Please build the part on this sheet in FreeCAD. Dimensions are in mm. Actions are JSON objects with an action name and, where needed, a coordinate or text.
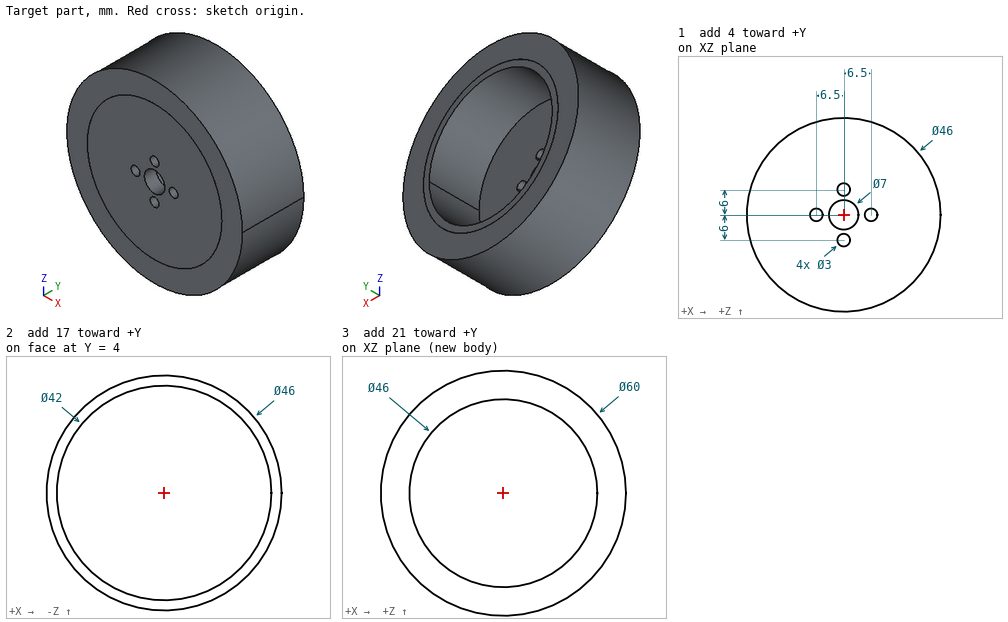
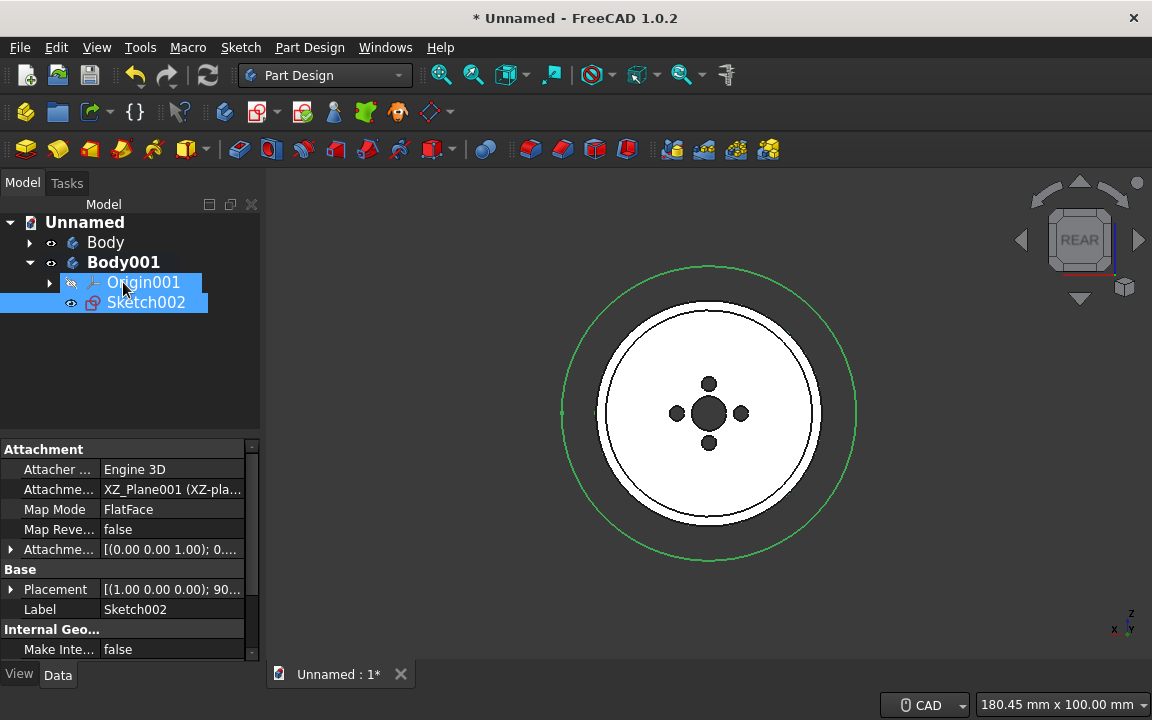
{"action": "left_click", "coordinate": [26, 150]}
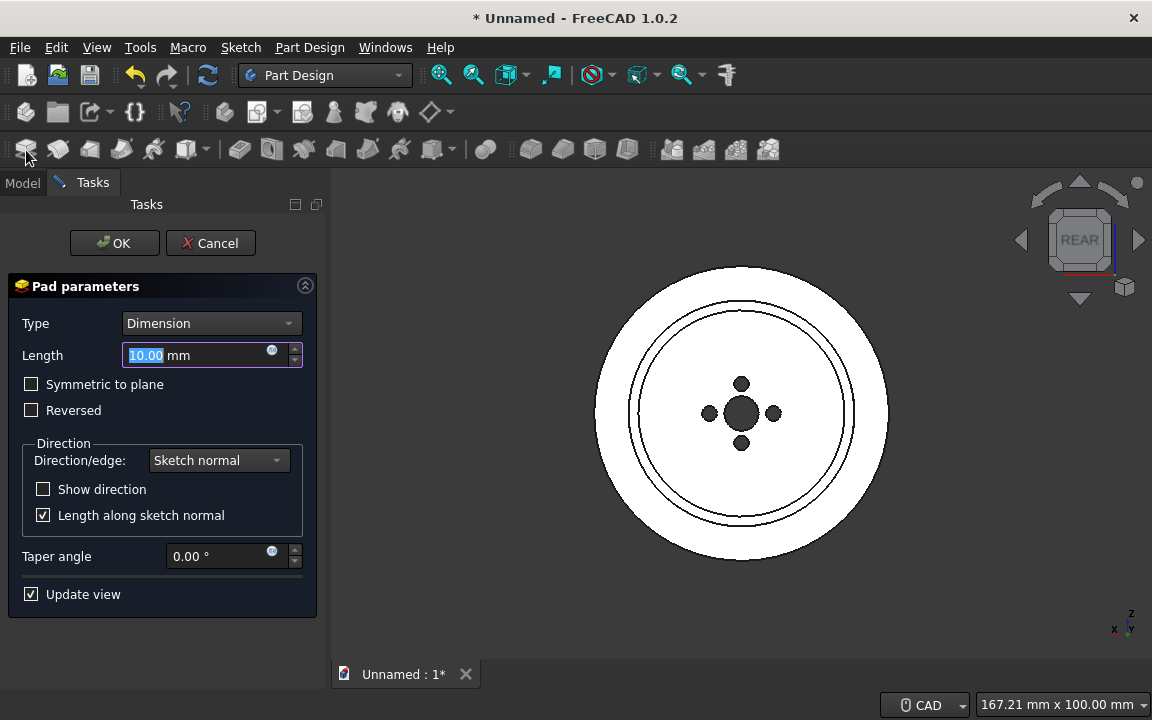
{"action": "type", "text": "21"}
{"action": "key", "text": "Tab"}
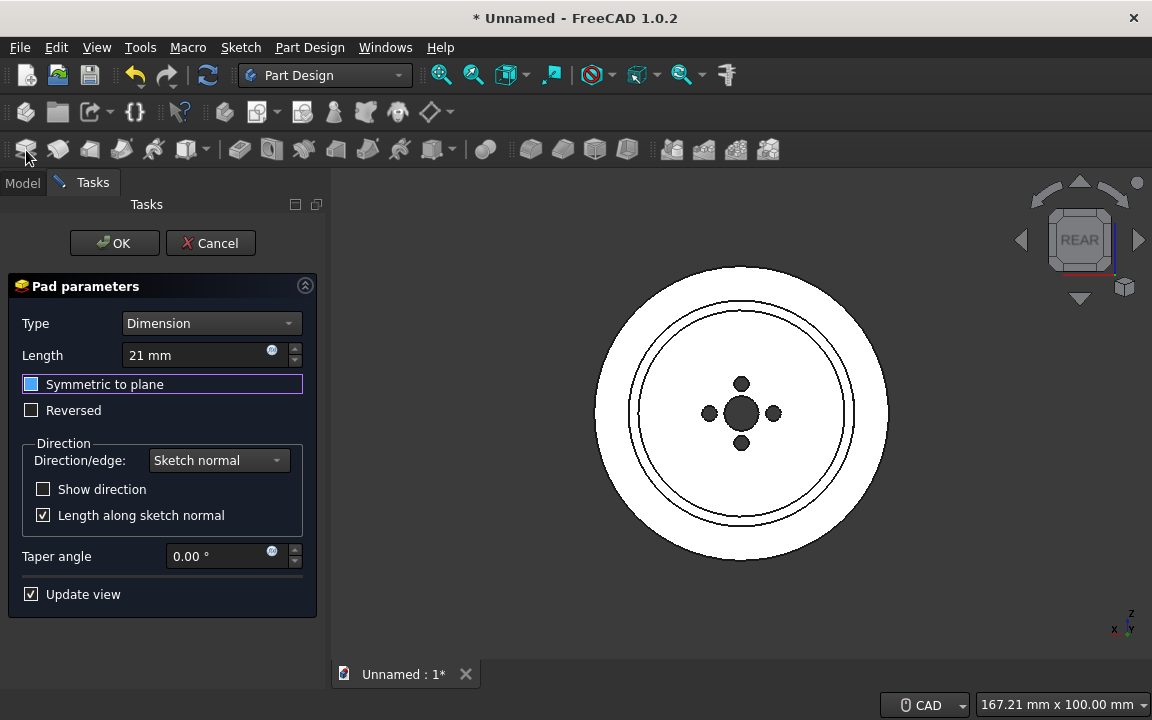
{"action": "left_click", "coordinate": [30, 410]}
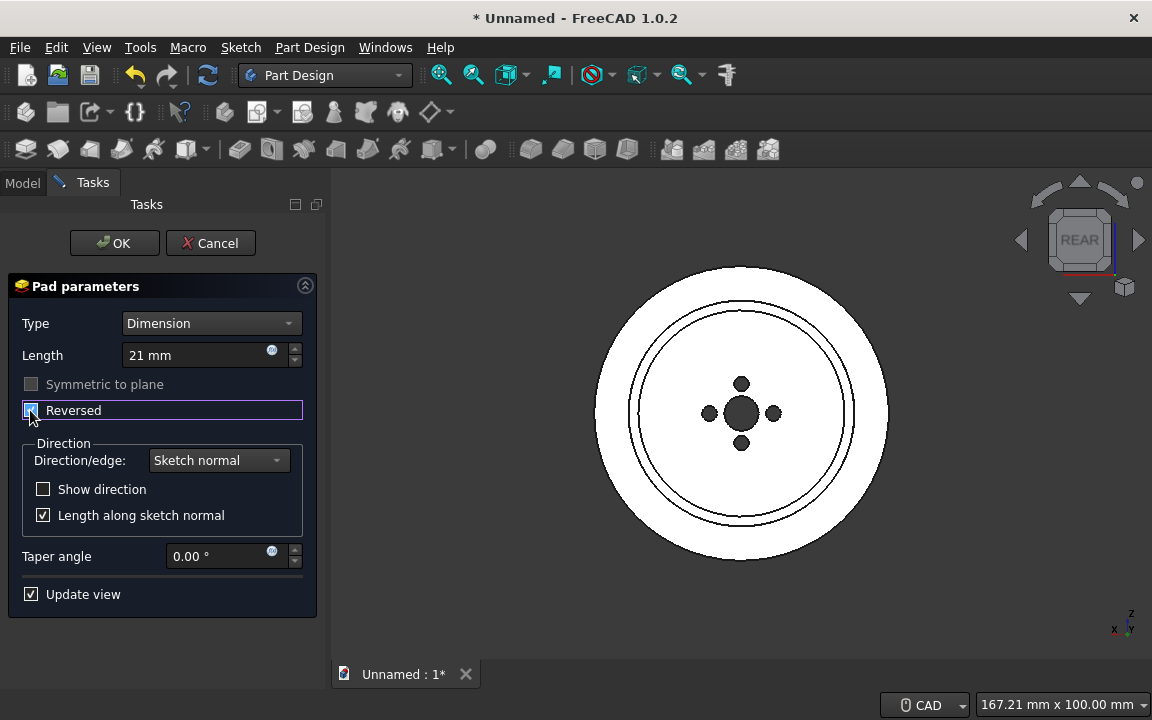
{"action": "left_click", "coordinate": [115, 243]}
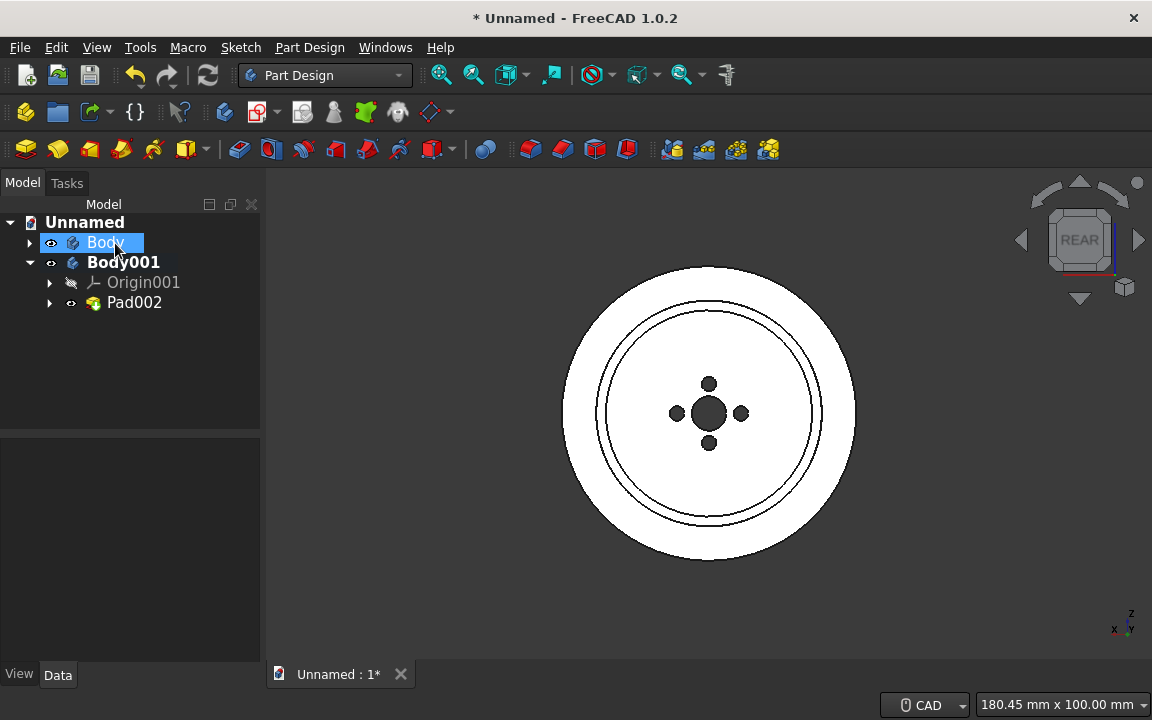
{"action": "key", "text": "0"}